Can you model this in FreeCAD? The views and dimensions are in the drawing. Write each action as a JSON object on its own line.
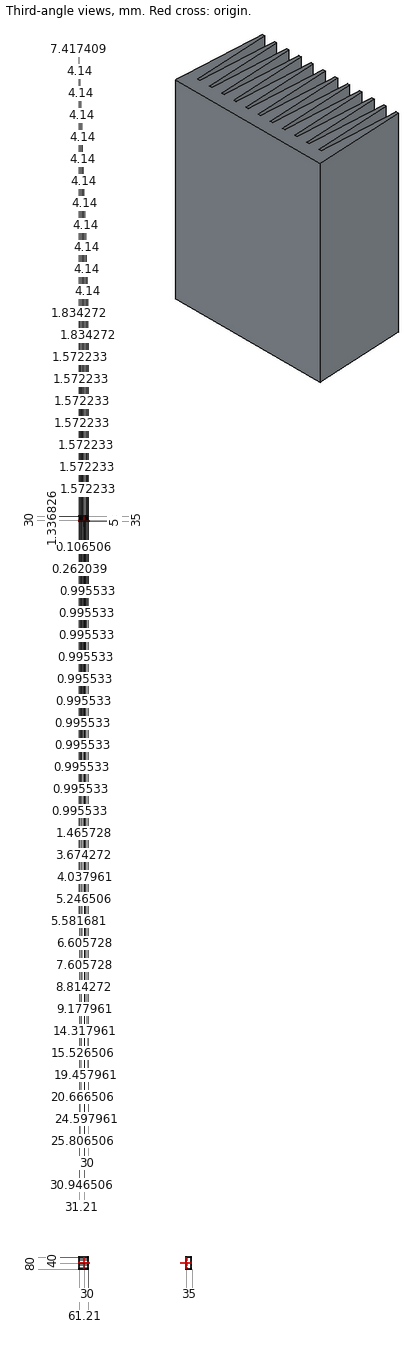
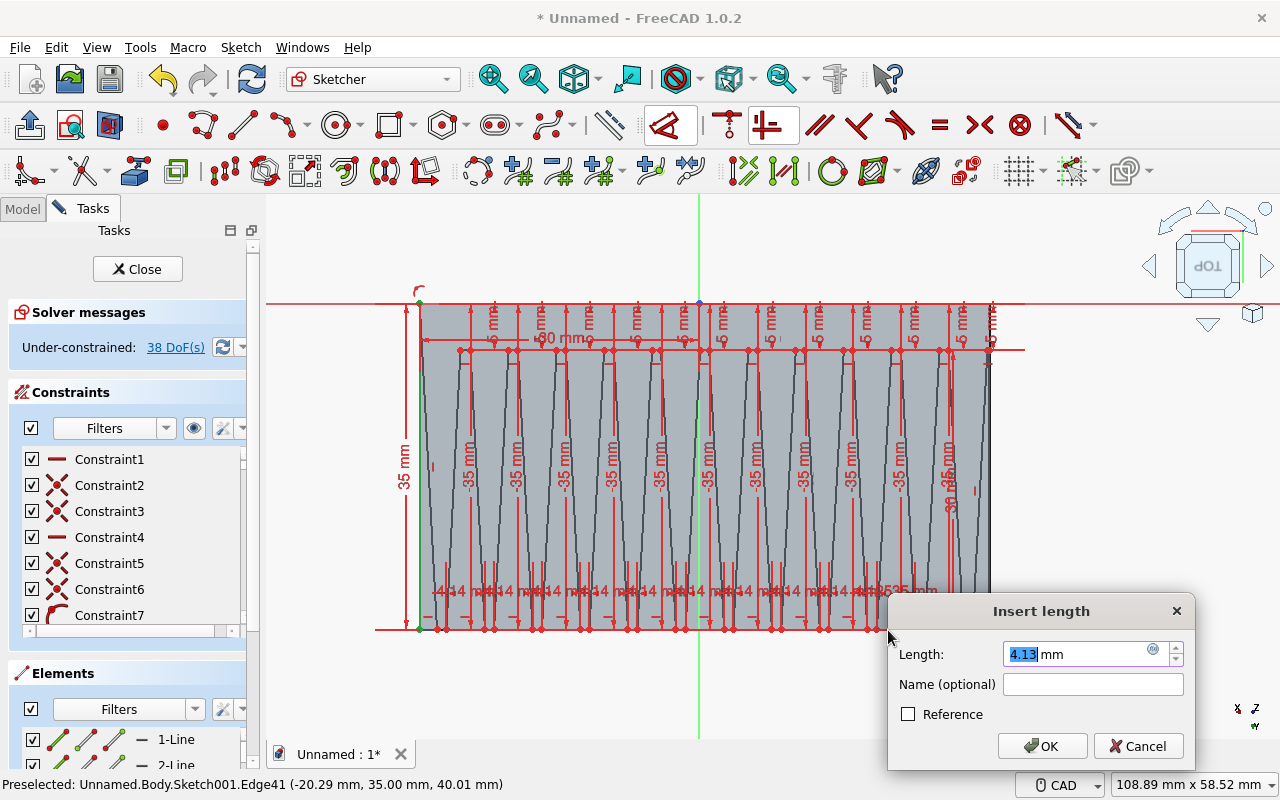
{"action": "type", "text": "4.14"}
{"action": "key", "text": "Return"}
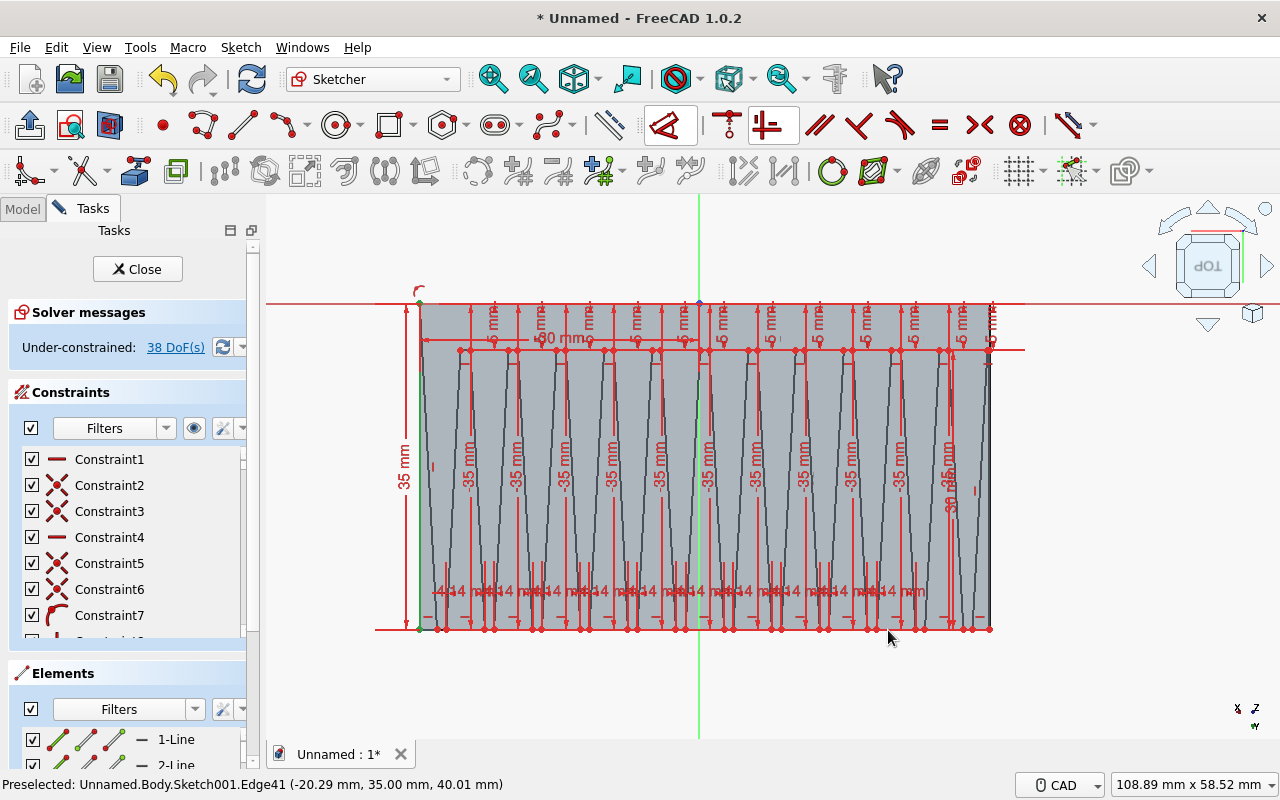
{"action": "left_click", "coordinate": [937, 630]}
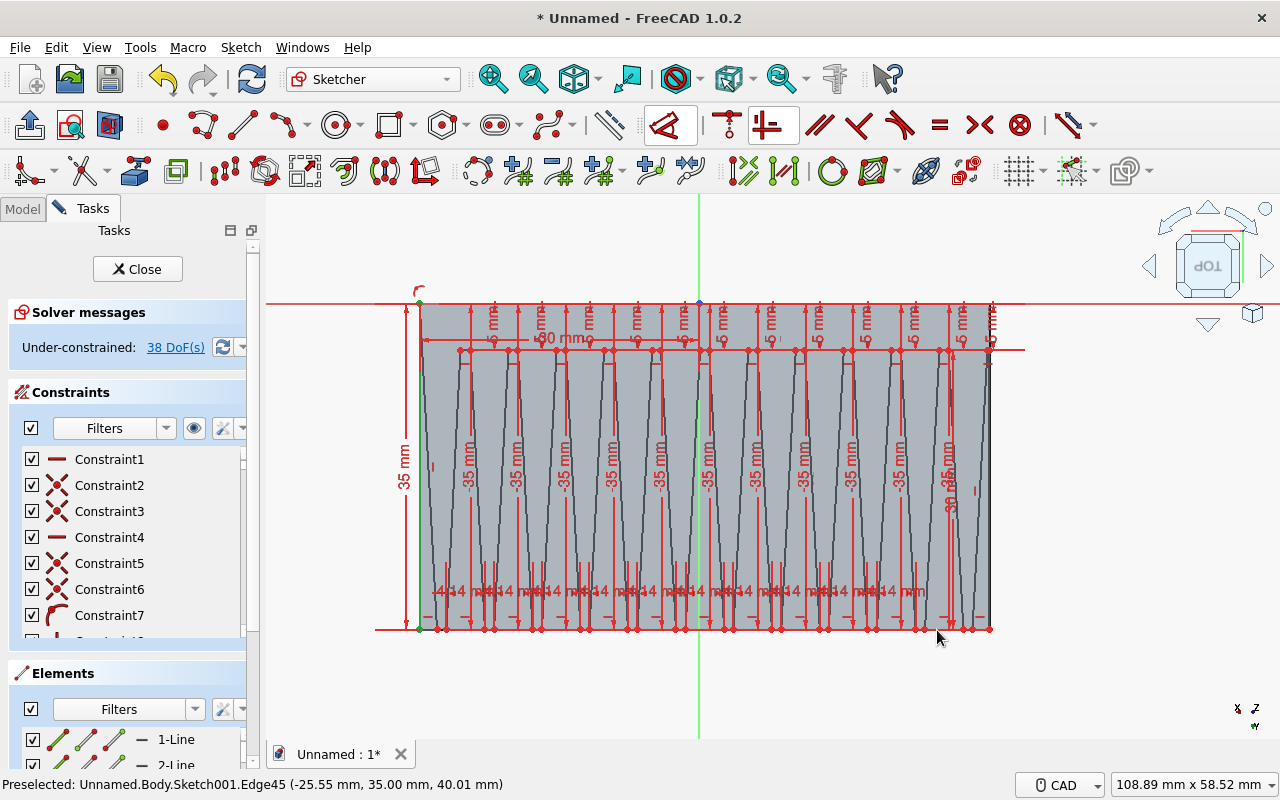
{"action": "left_click", "coordinate": [692, 126]}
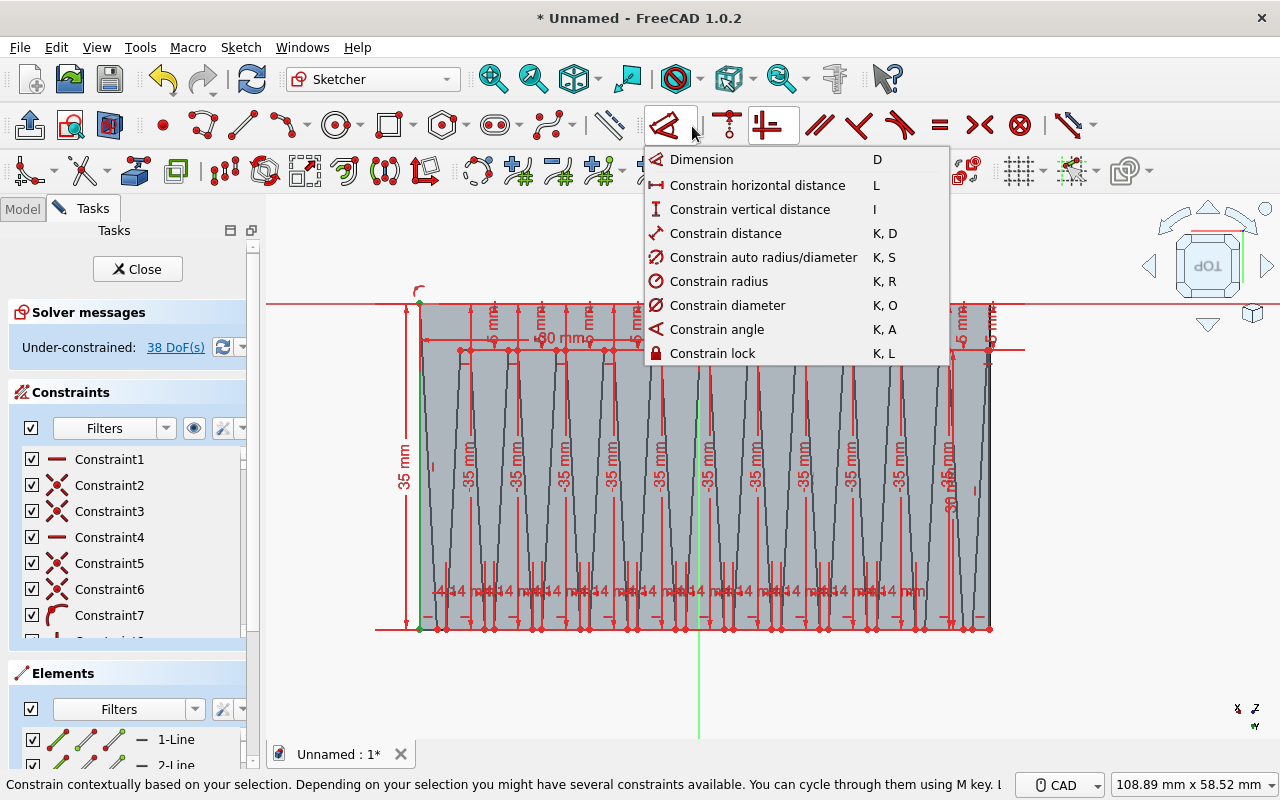
{"action": "left_click", "coordinate": [797, 185]}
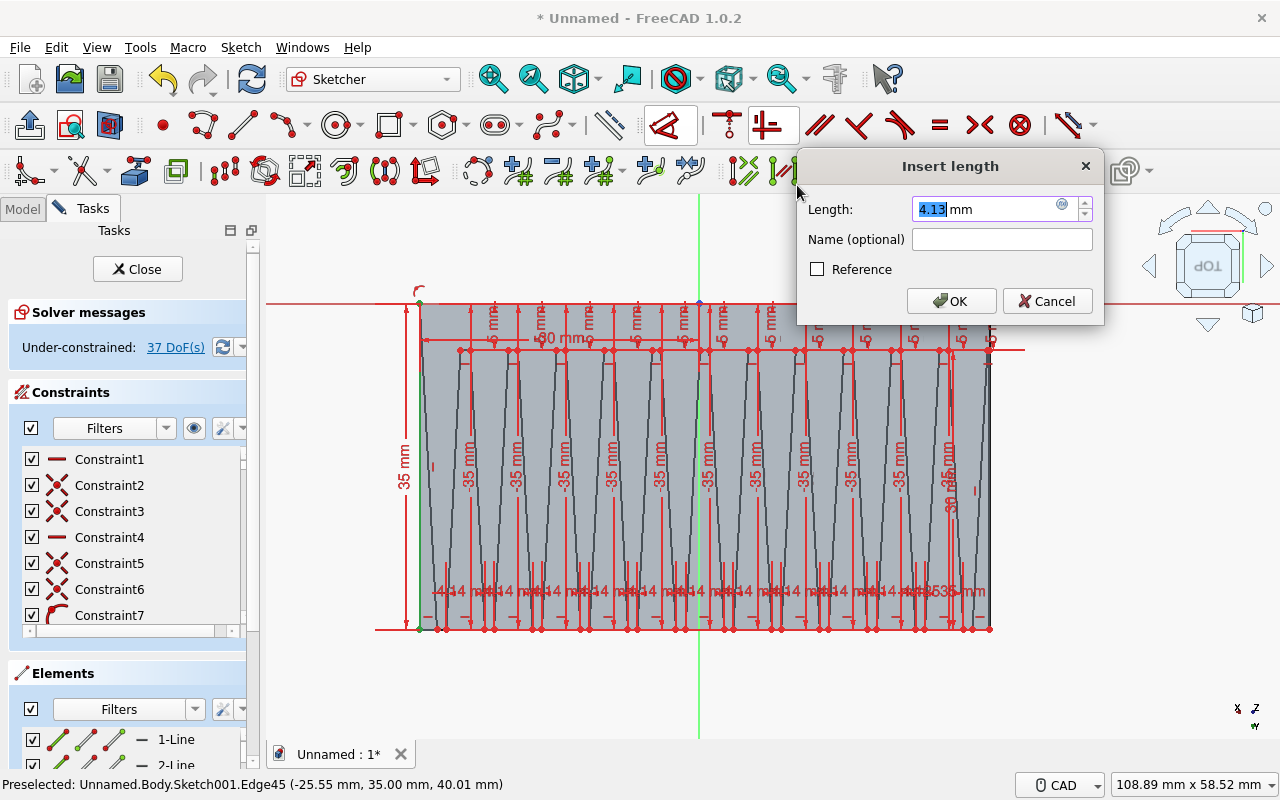
{"action": "type", "text": "4.14"}
{"action": "key", "text": "Return"}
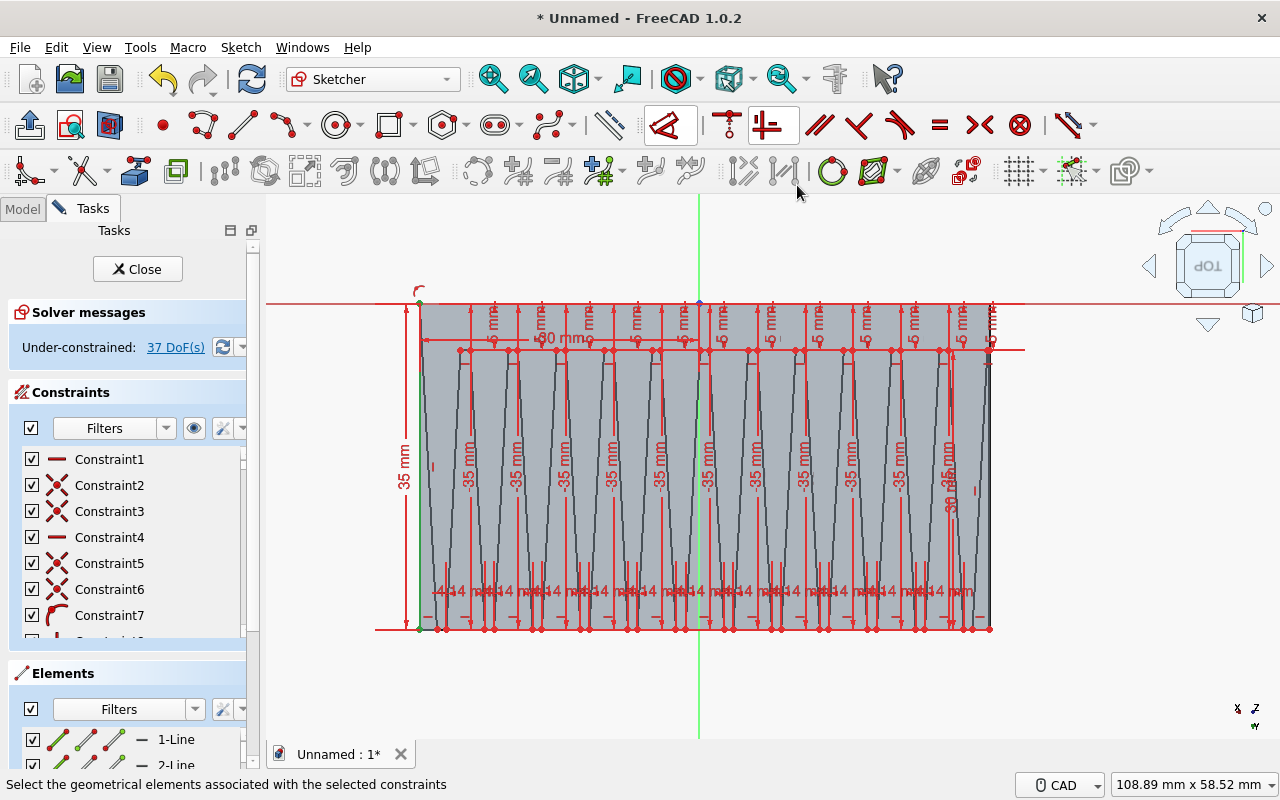
{"action": "scroll", "coordinate": [465, 350], "scroll_direction": "up", "scroll_amount": 8}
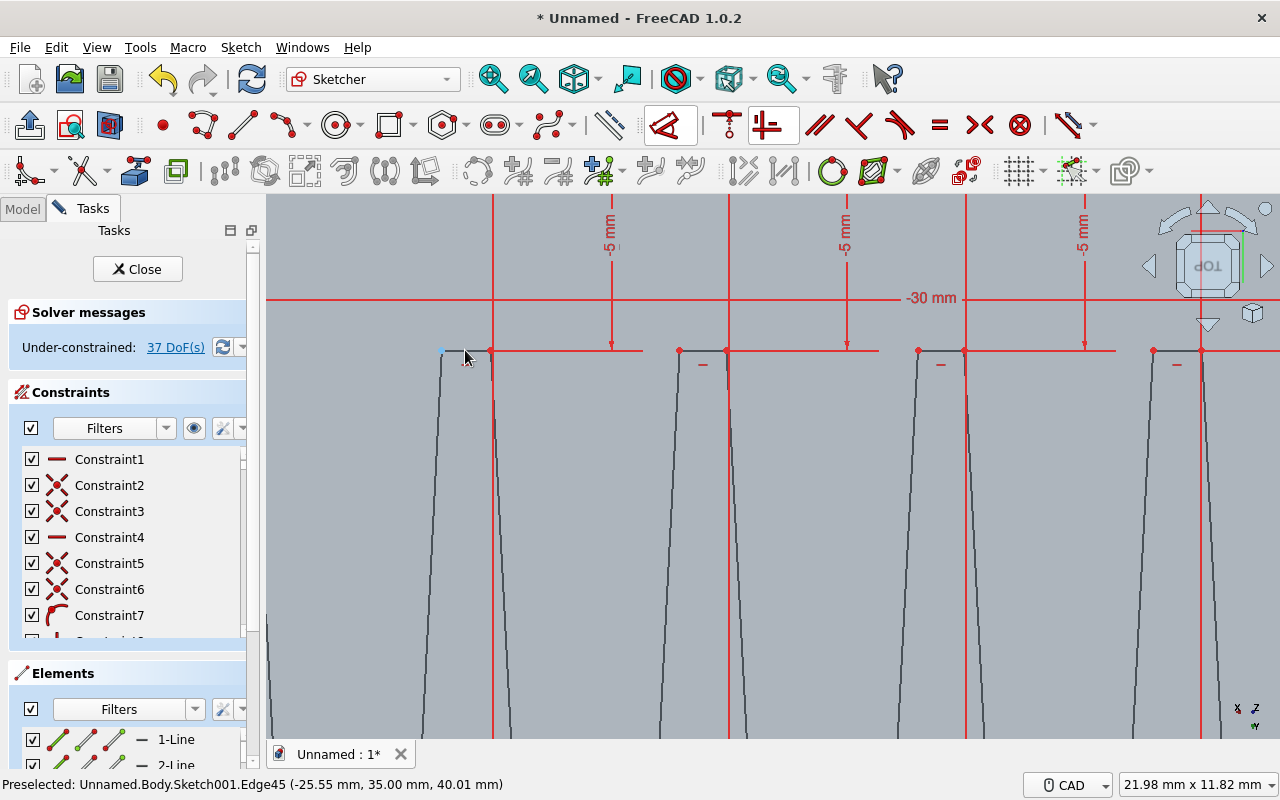
{"action": "left_click", "coordinate": [466, 351]}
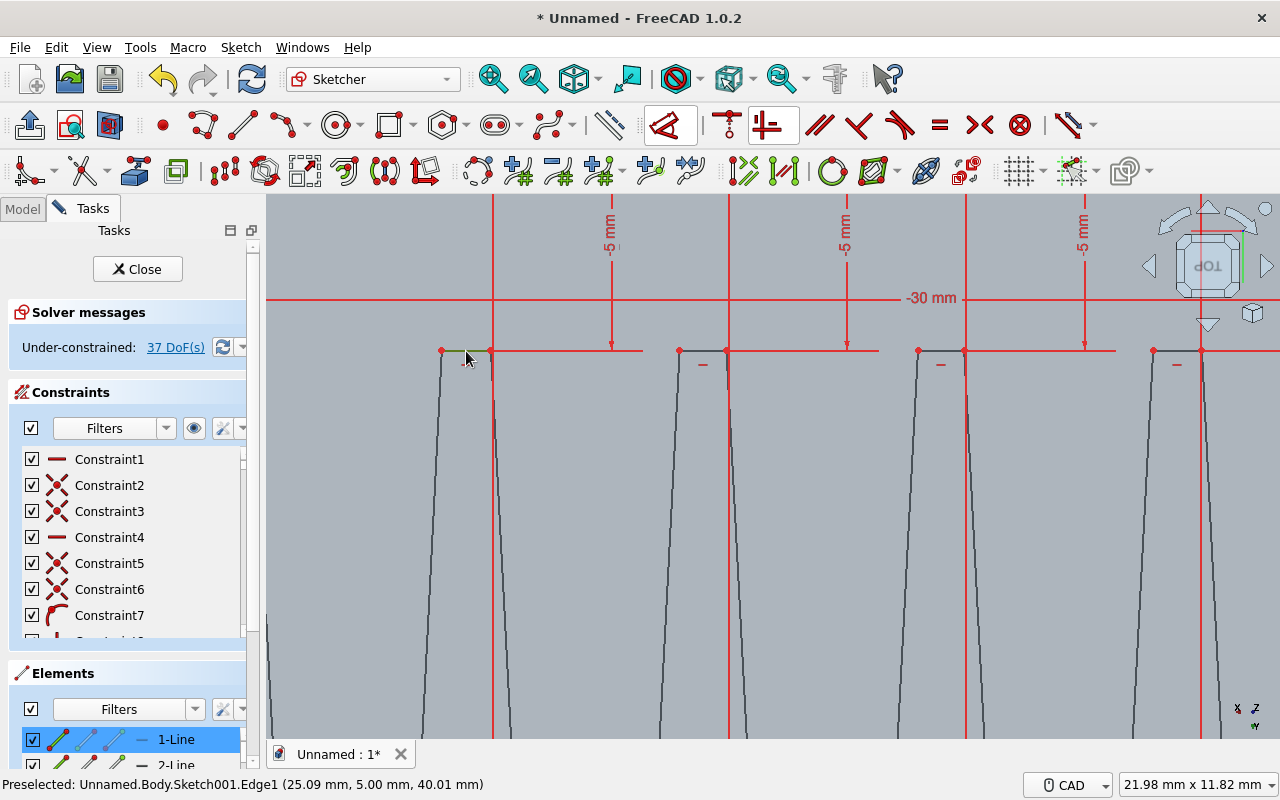
{"action": "key", "text": "l"}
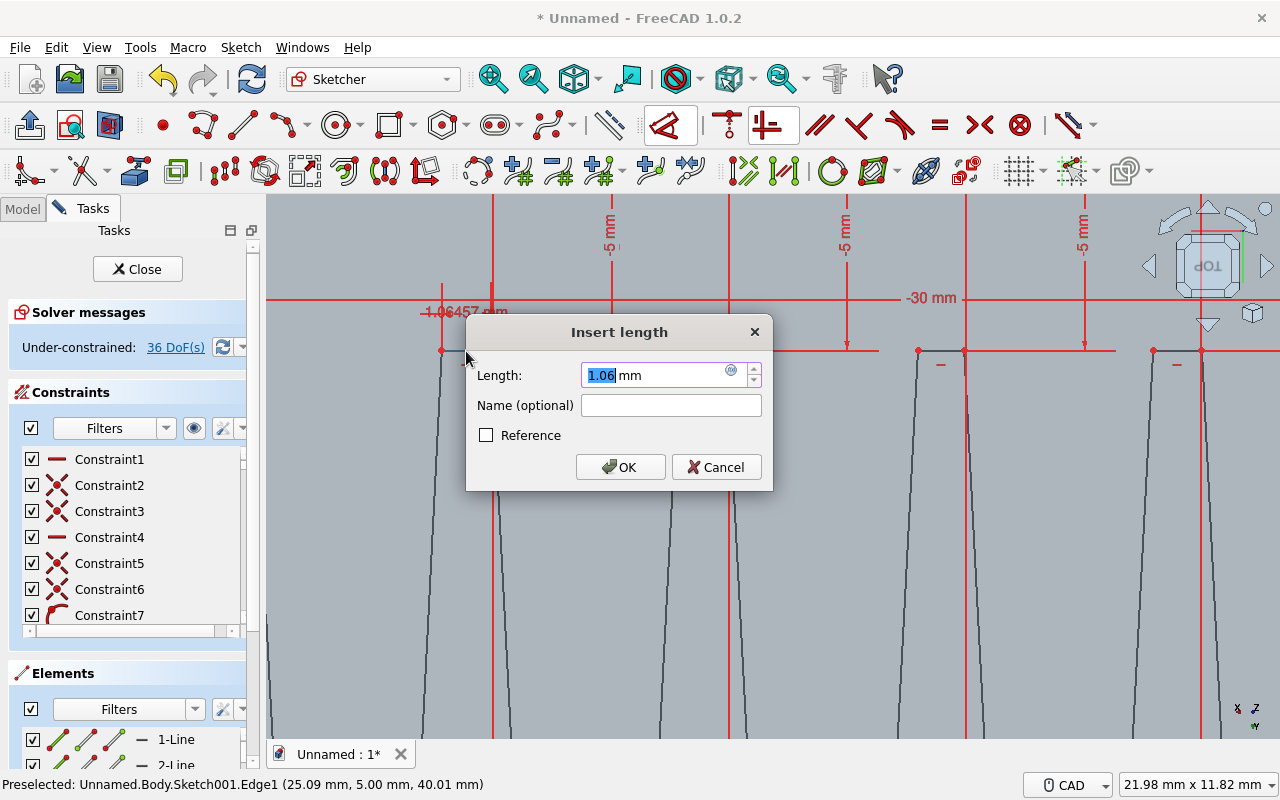
{"action": "type", "text": "0.995533"}
{"action": "key", "text": "Return"}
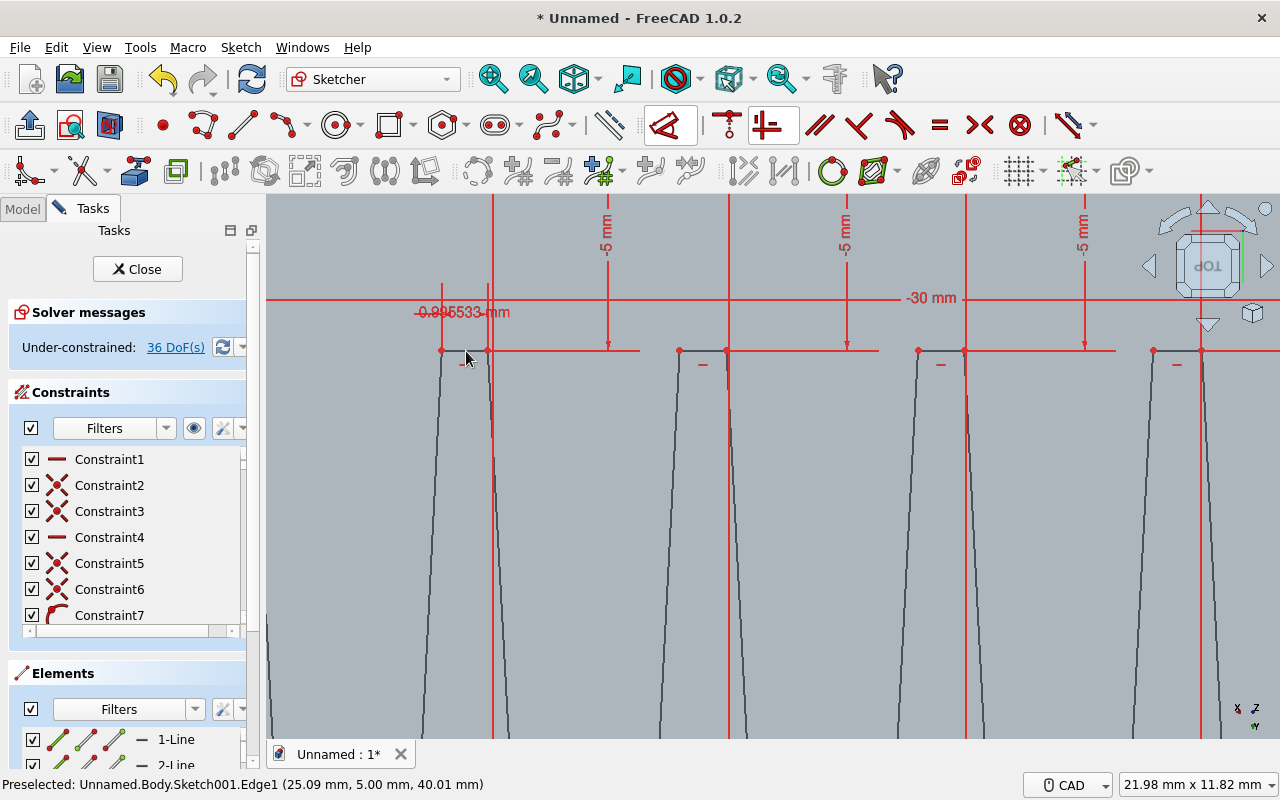
{"action": "scroll", "coordinate": [465, 350], "scroll_direction": "down", "scroll_amount": 8}